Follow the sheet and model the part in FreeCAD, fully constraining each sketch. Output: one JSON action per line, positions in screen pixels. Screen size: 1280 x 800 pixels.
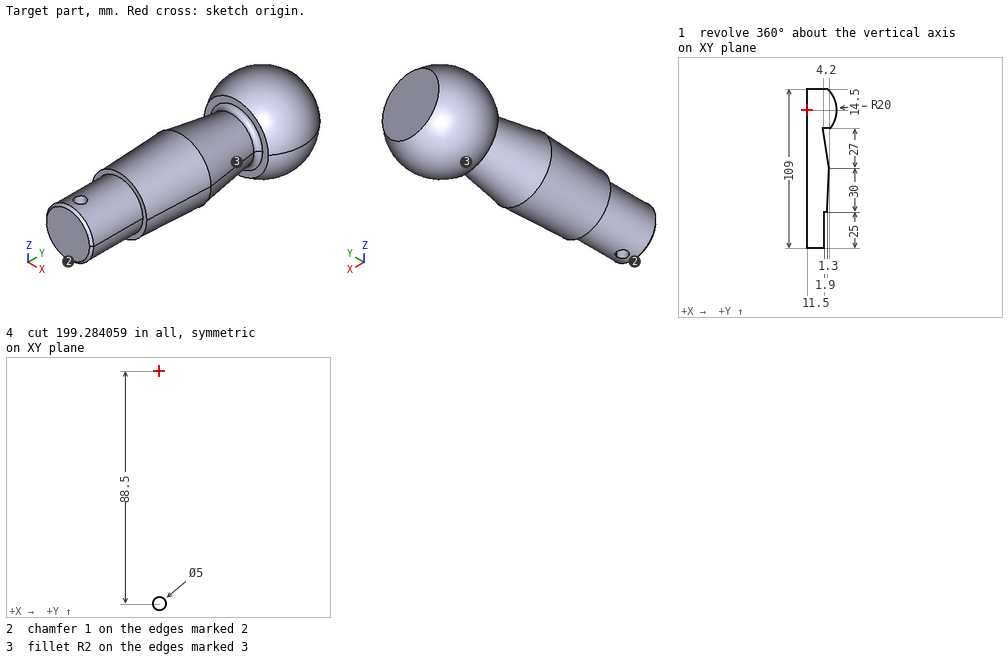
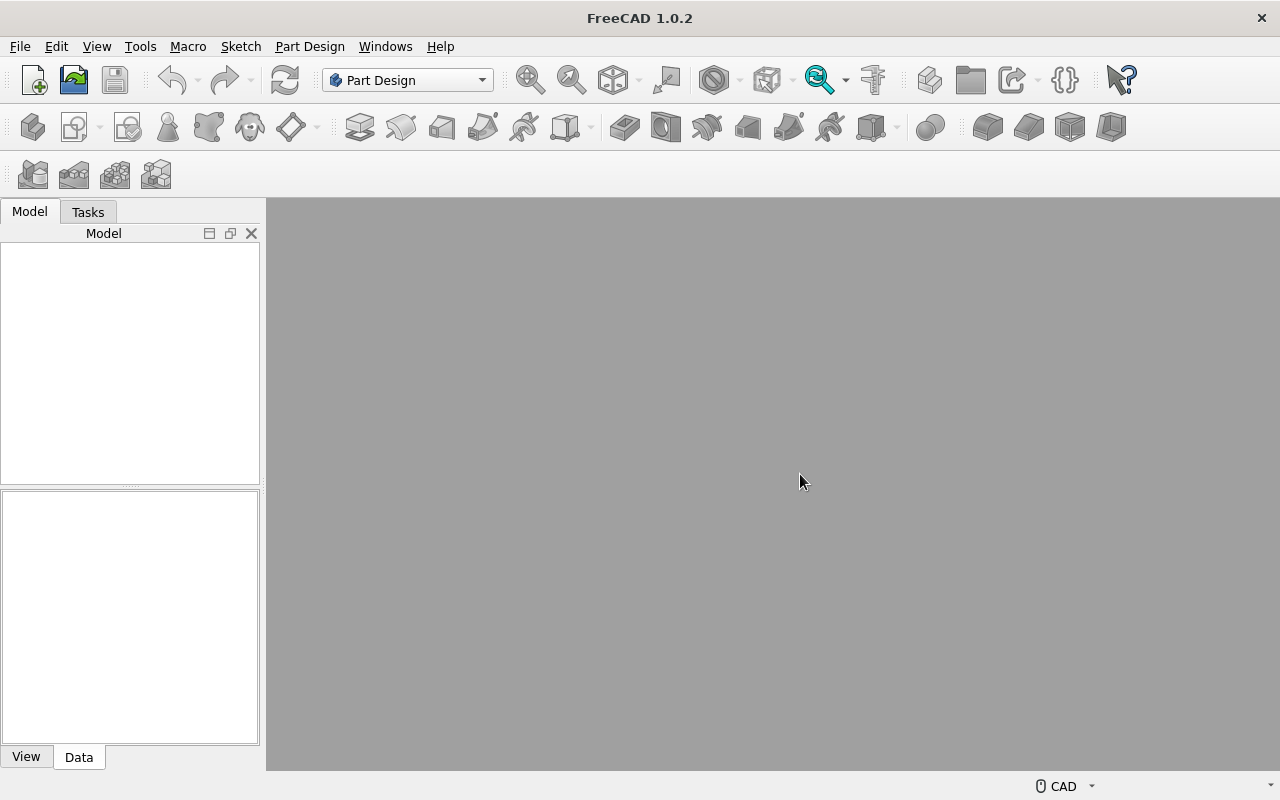
{"action": "key", "text": "ctrl+n"}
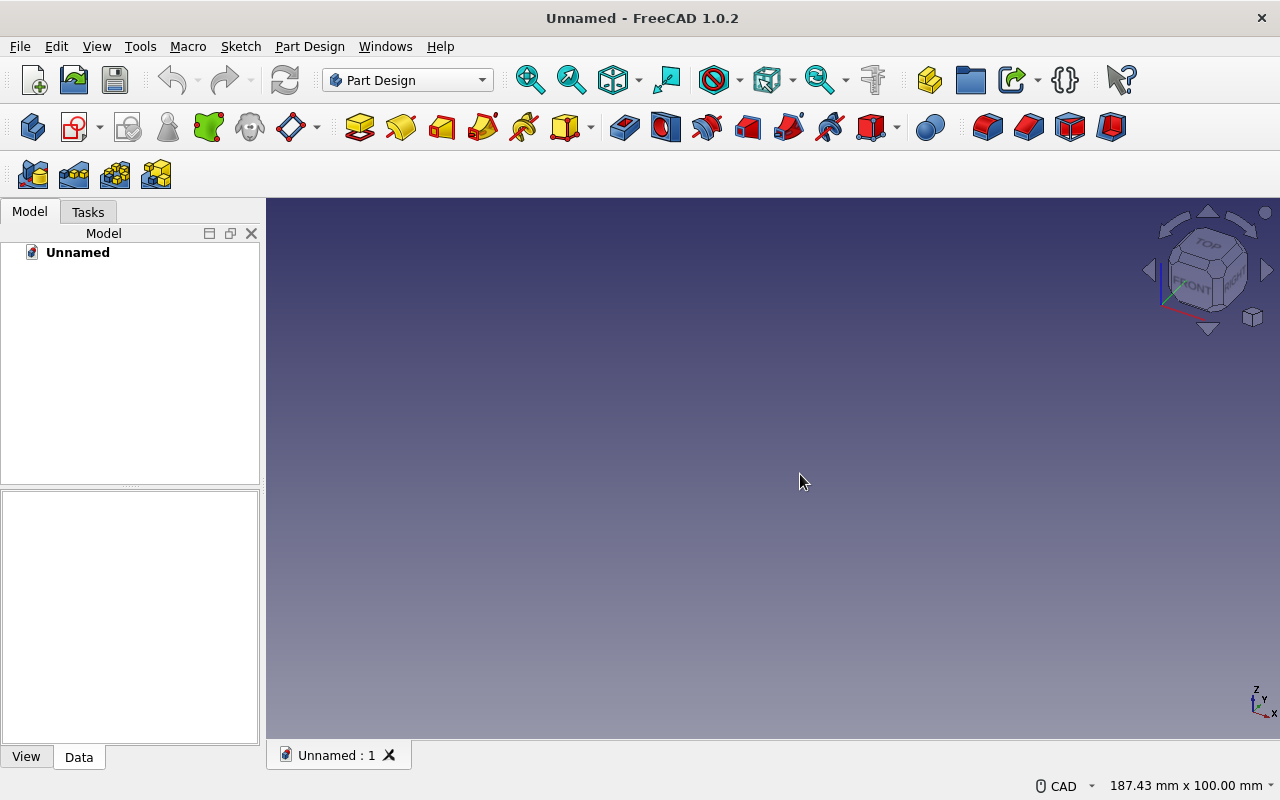
{"action": "left_click", "coordinate": [74, 128]}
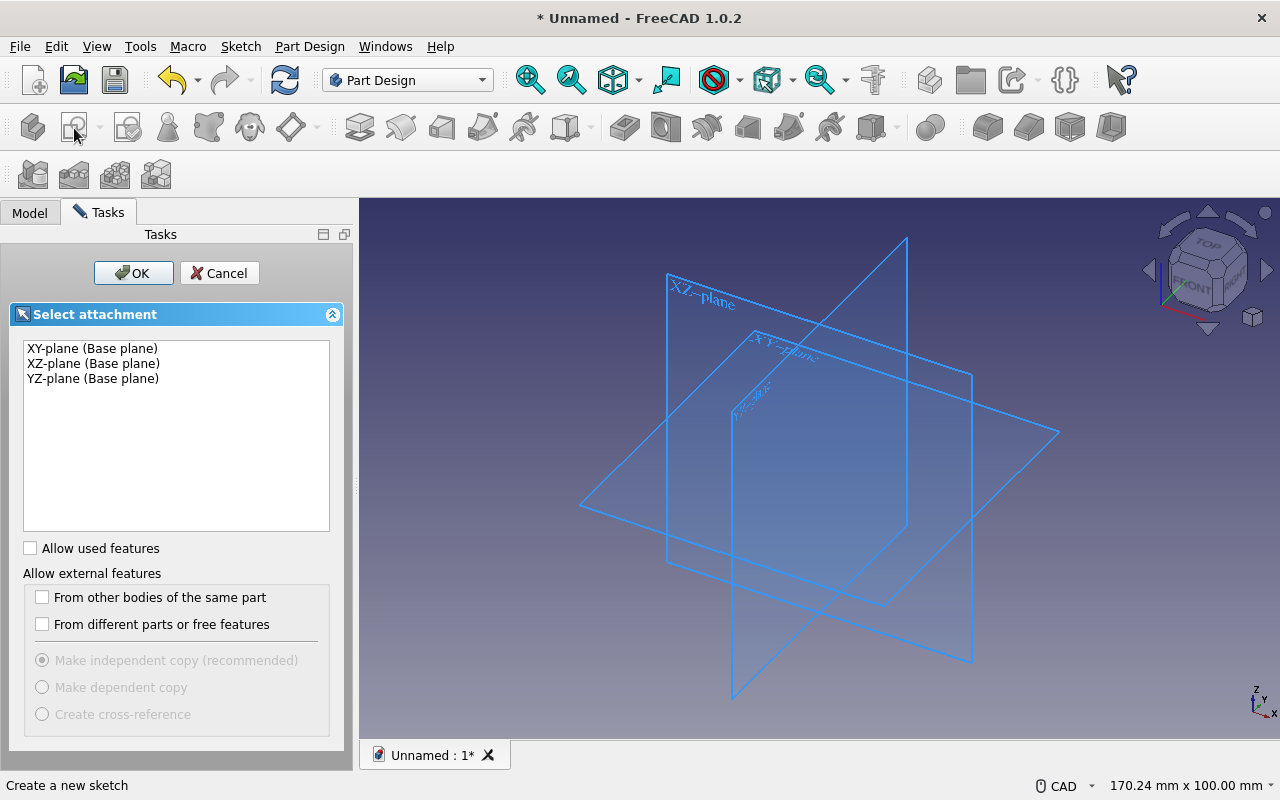
{"action": "left_click", "coordinate": [84, 348]}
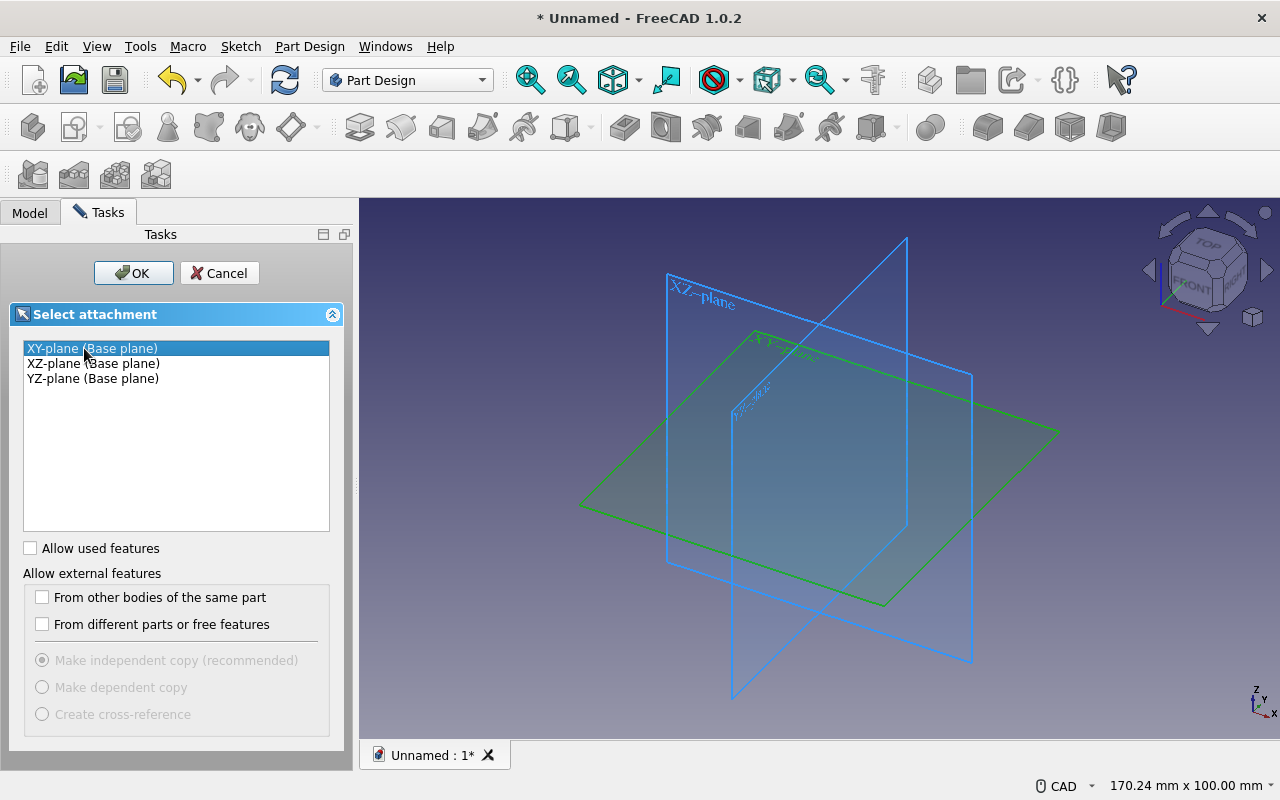
{"action": "left_click", "coordinate": [134, 273]}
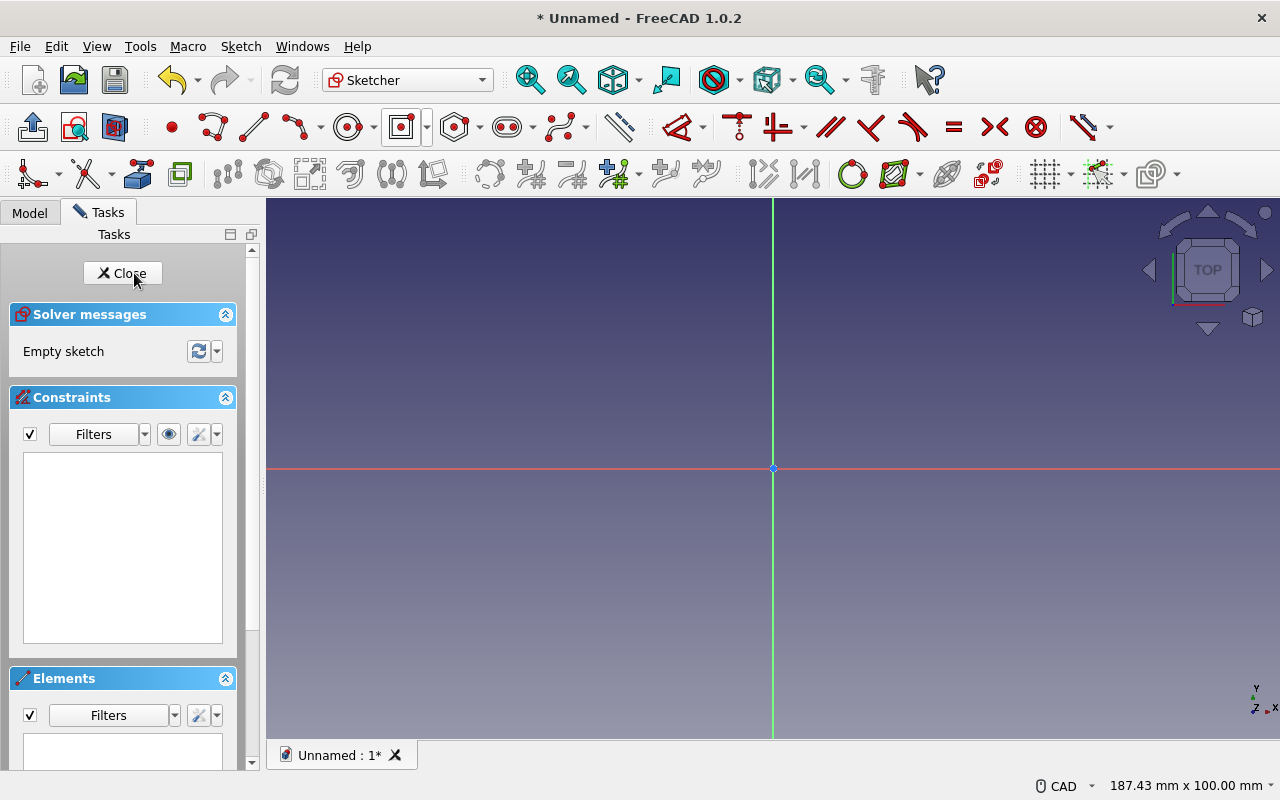
{"action": "scroll", "coordinate": [556, 226], "scroll_direction": "down", "scroll_amount": 3}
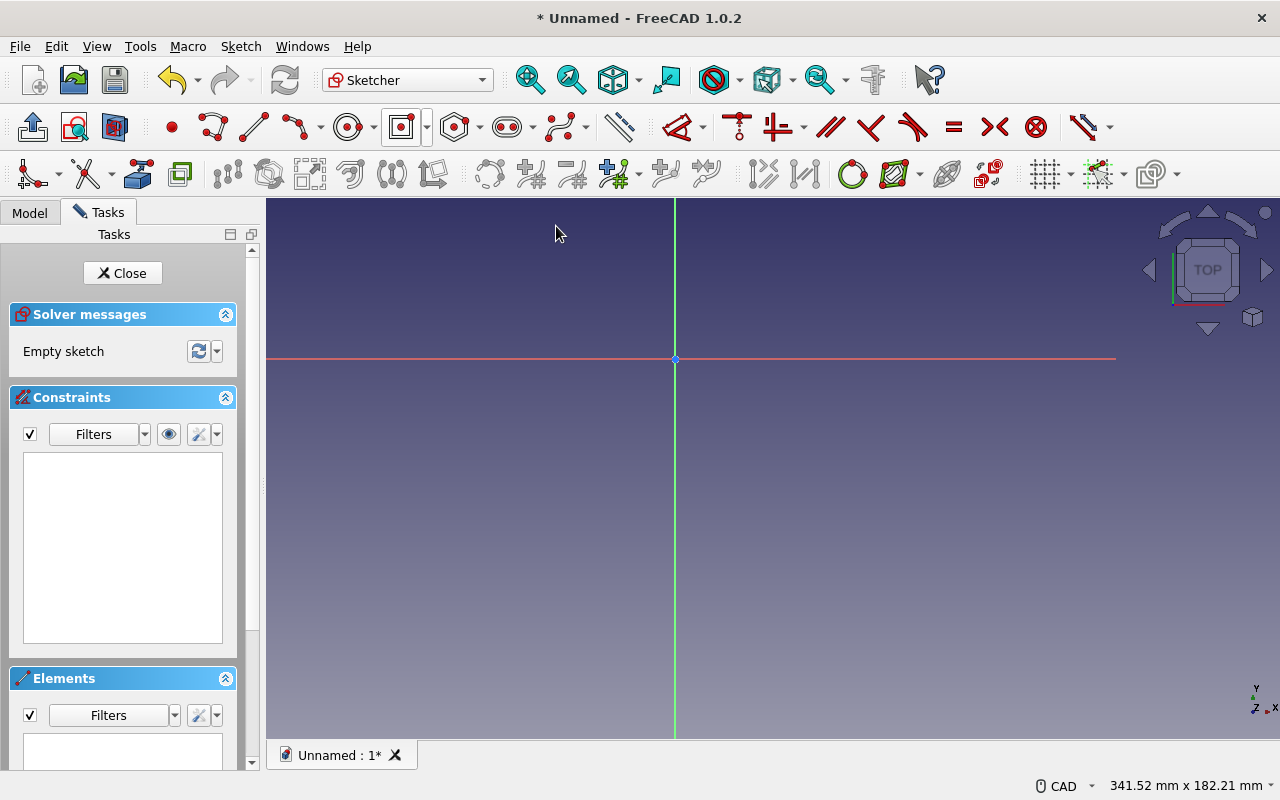
{"action": "left_click", "coordinate": [213, 128]}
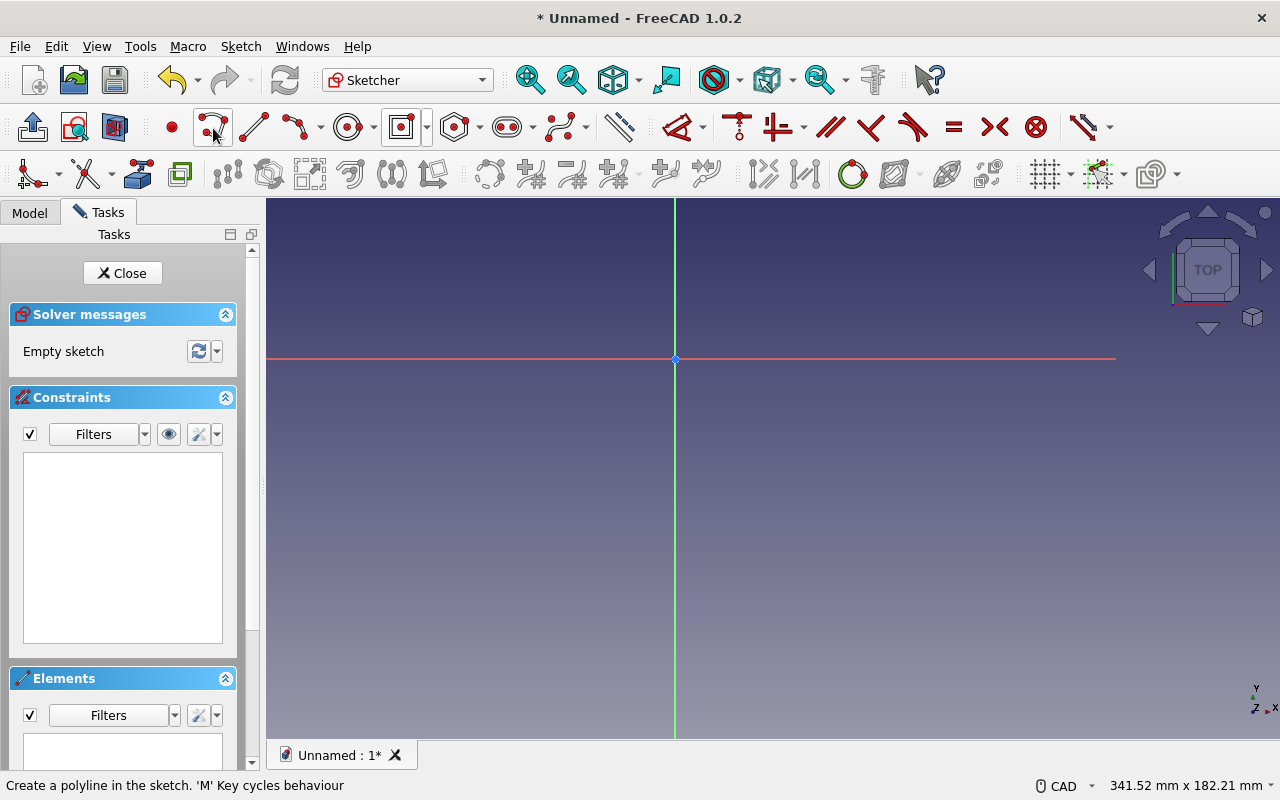
{"action": "left_click", "coordinate": [716, 316]}
{"action": "left_click", "coordinate": [675, 316]}
{"action": "left_click", "coordinate": [684, 640]}
{"action": "left_click", "coordinate": [709, 640]}
{"action": "left_click", "coordinate": [709, 565]}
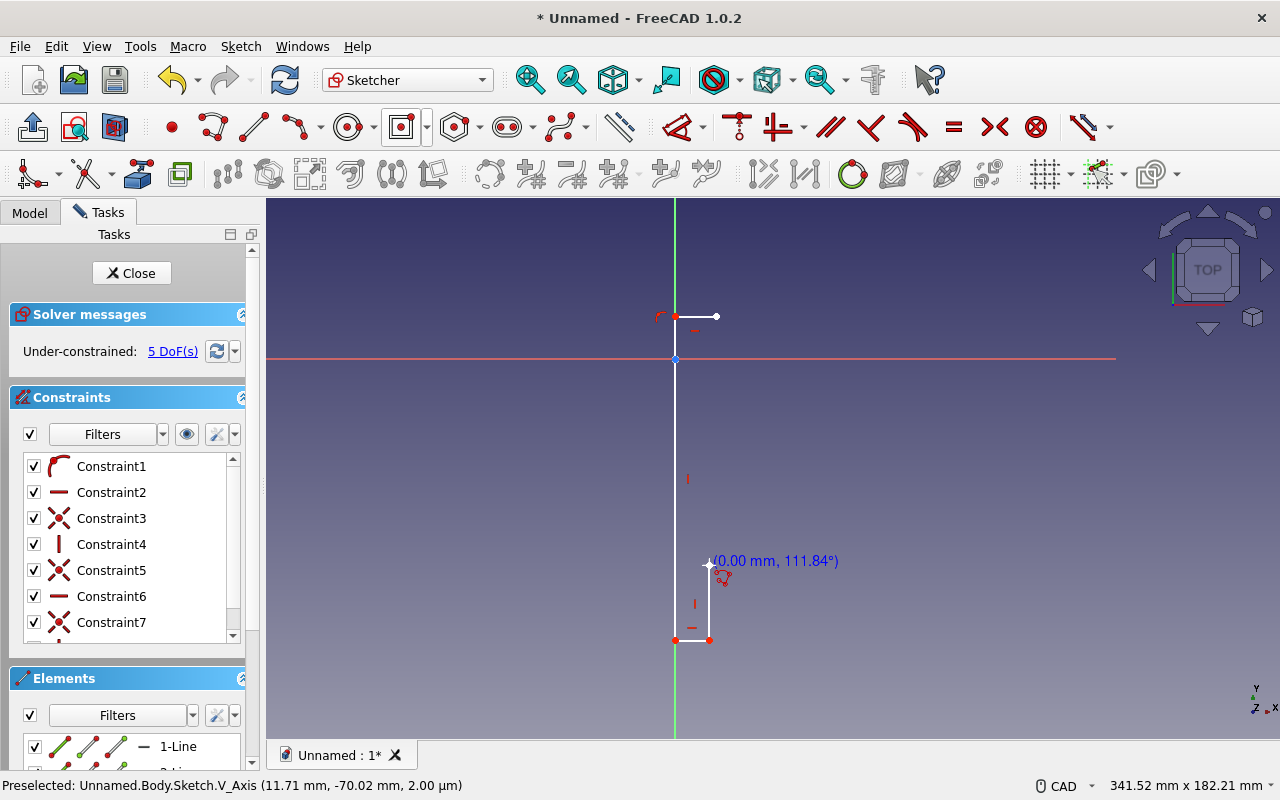
{"action": "scroll", "coordinate": [715, 565], "scroll_direction": "up", "scroll_amount": 6}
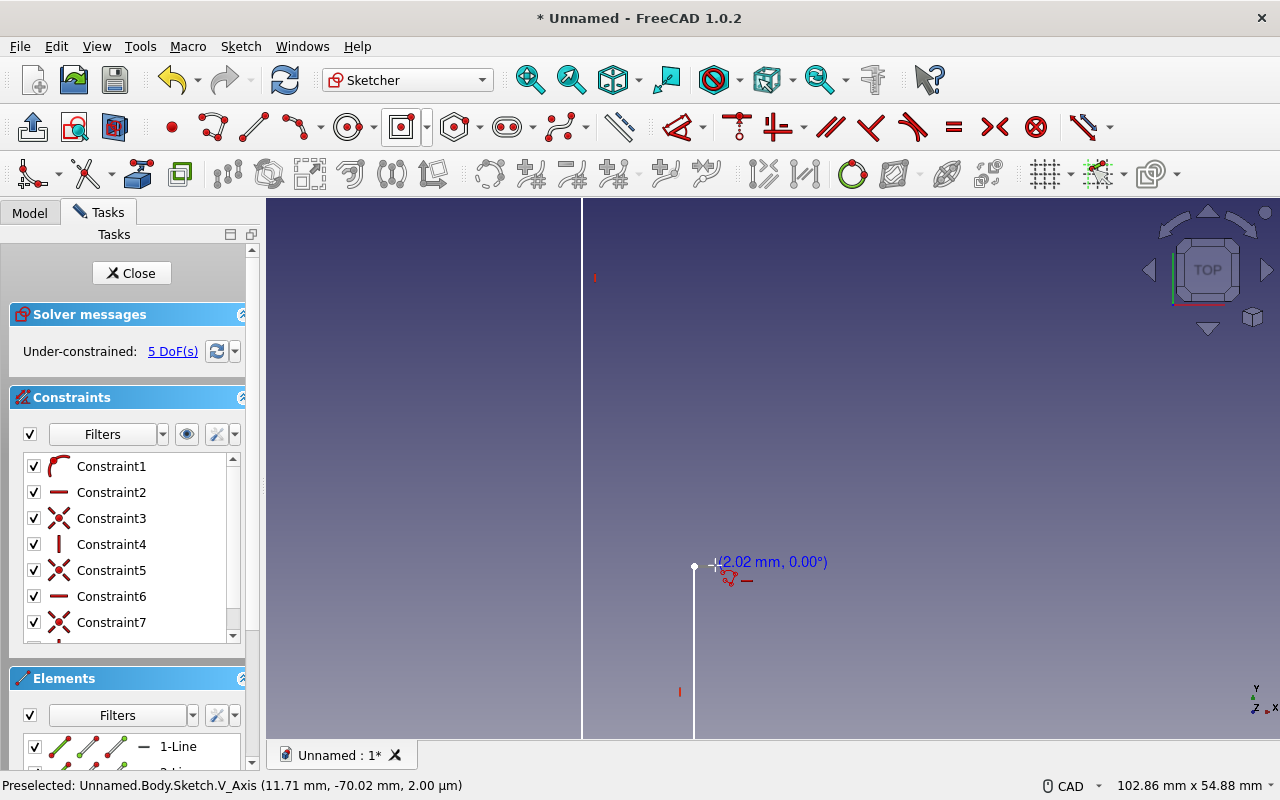
{"action": "left_click", "coordinate": [714, 563]}
{"action": "left_click", "coordinate": [729, 269]}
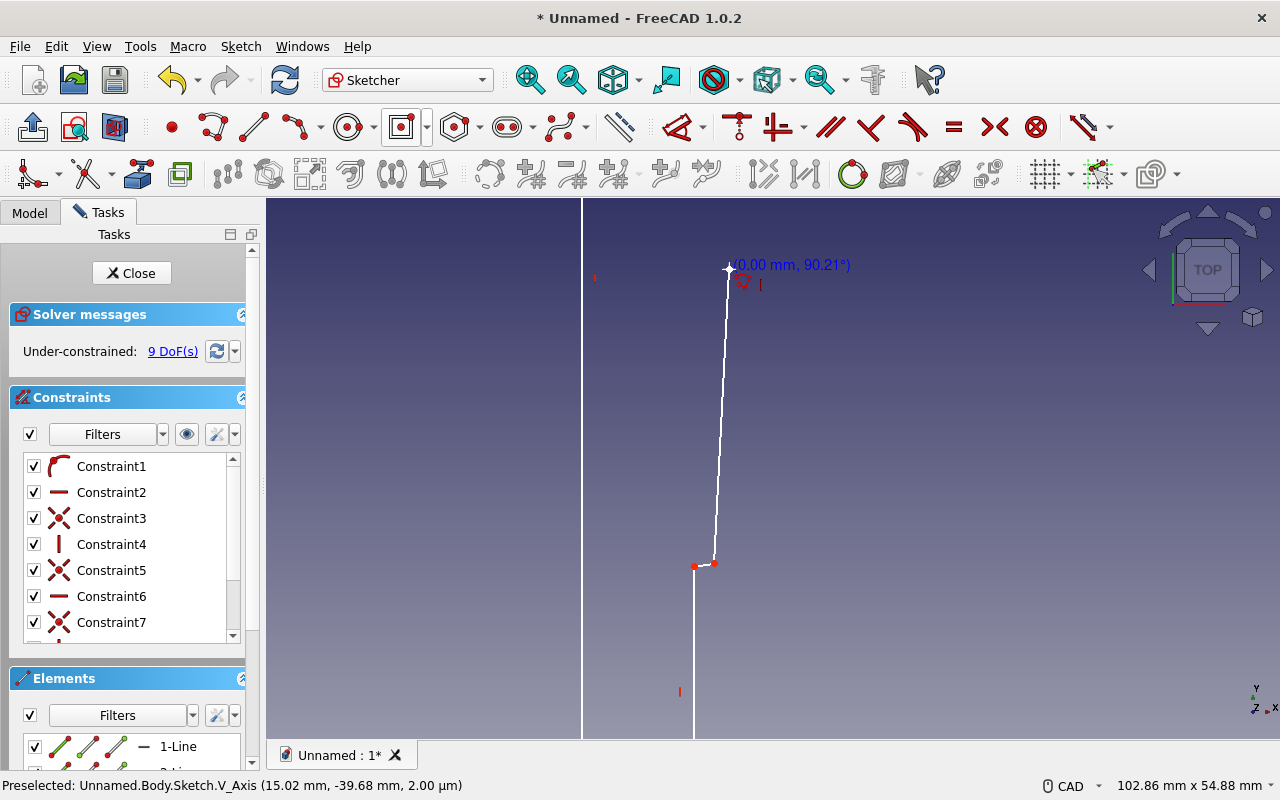
{"action": "scroll", "coordinate": [715, 552], "scroll_direction": "down", "scroll_amount": 6}